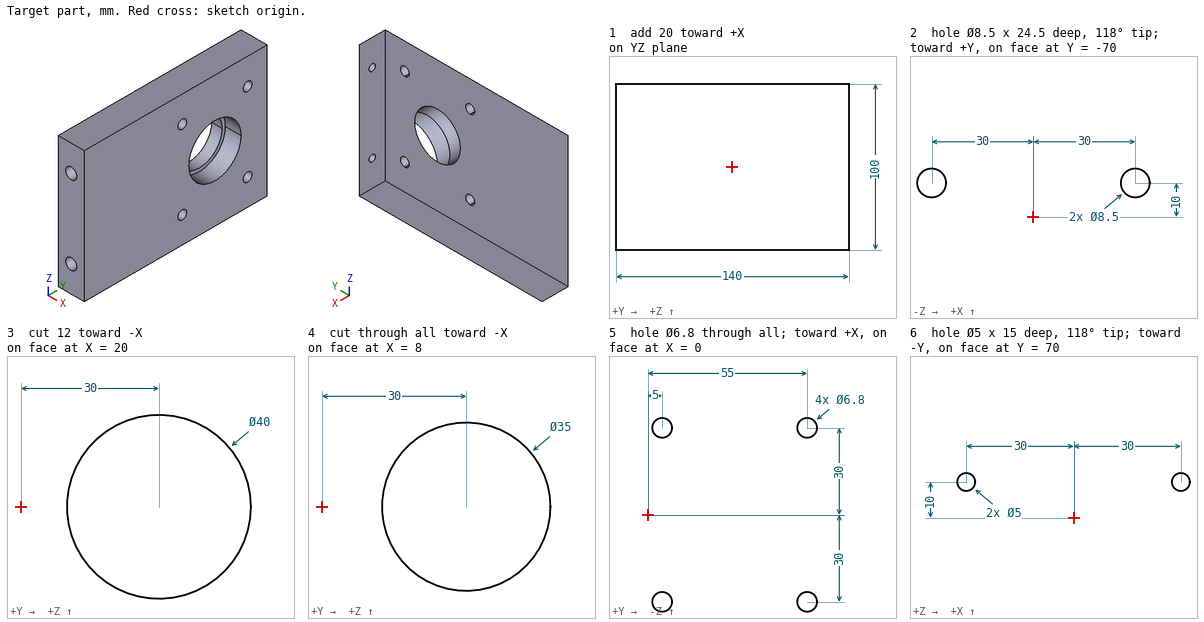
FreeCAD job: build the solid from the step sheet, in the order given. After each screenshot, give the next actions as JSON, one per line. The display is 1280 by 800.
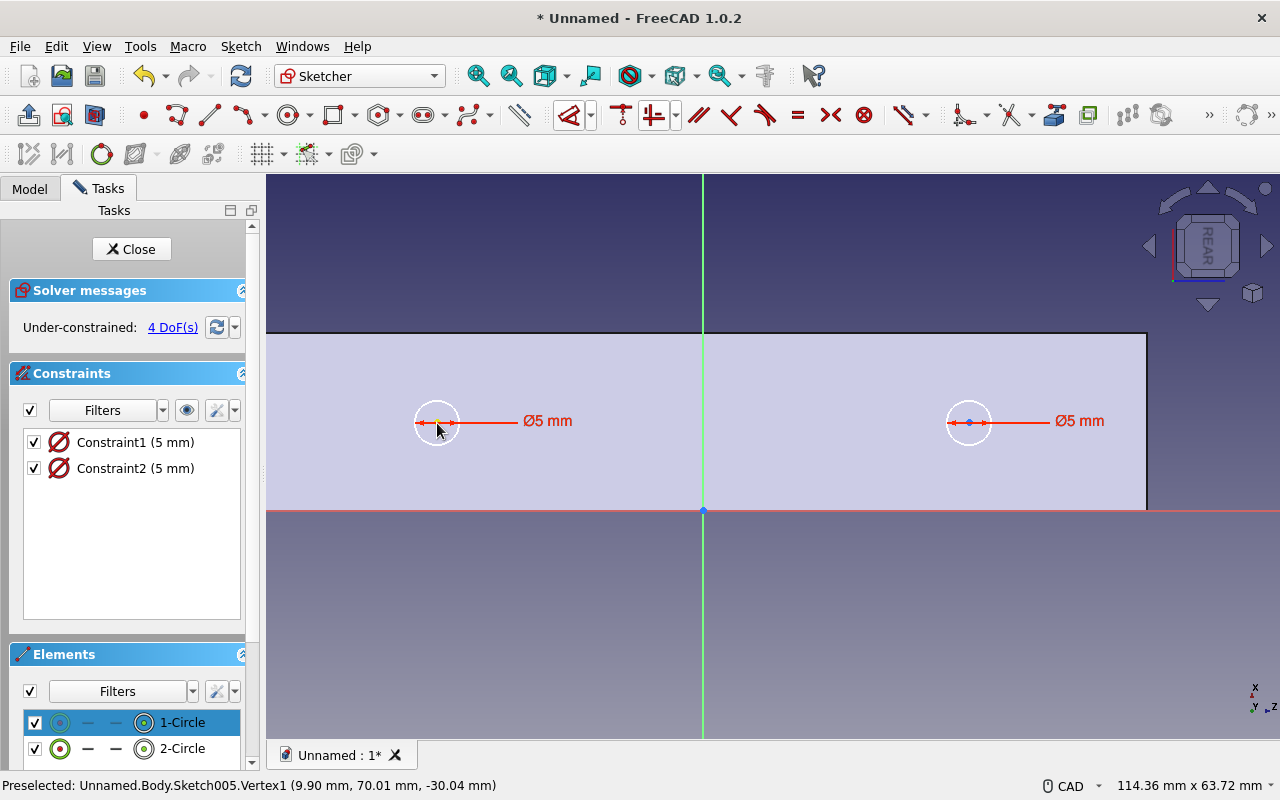
{"action": "left_click", "coordinate": [969, 423]}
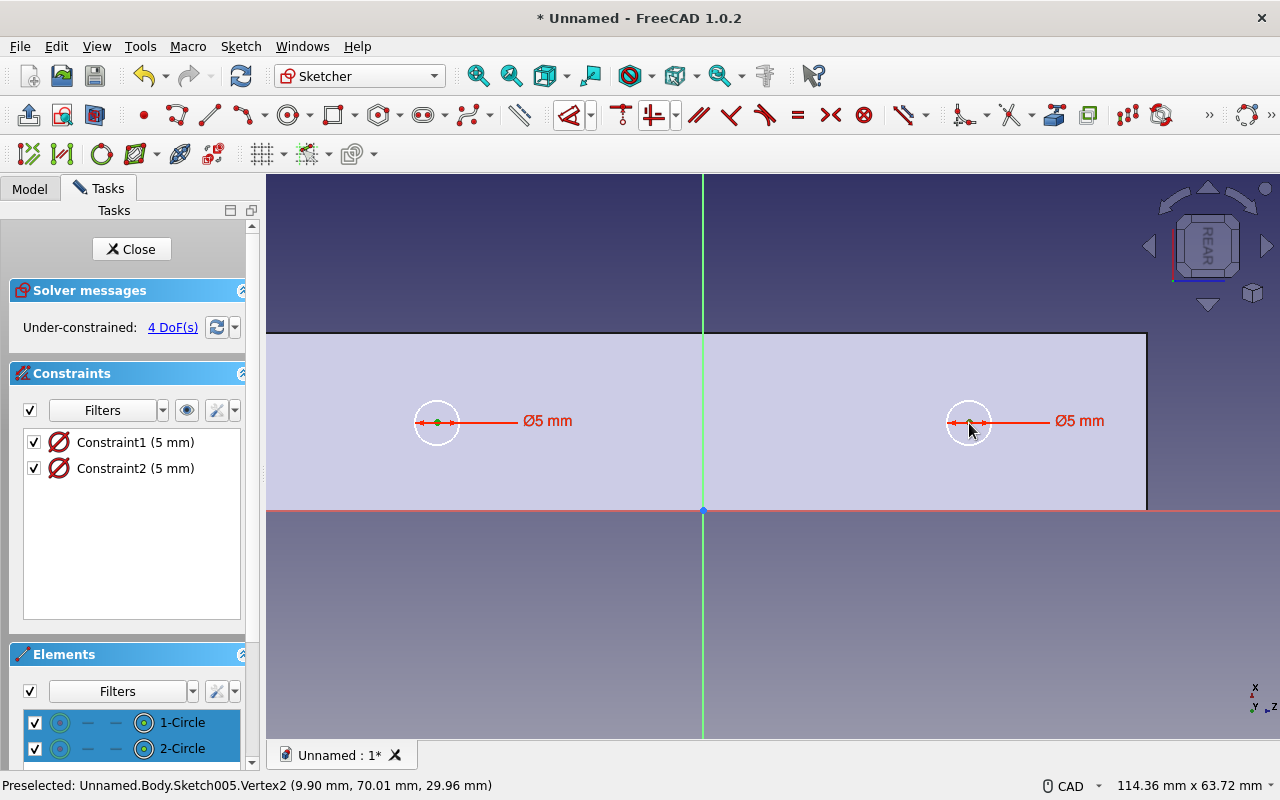
{"action": "key", "text": "h"}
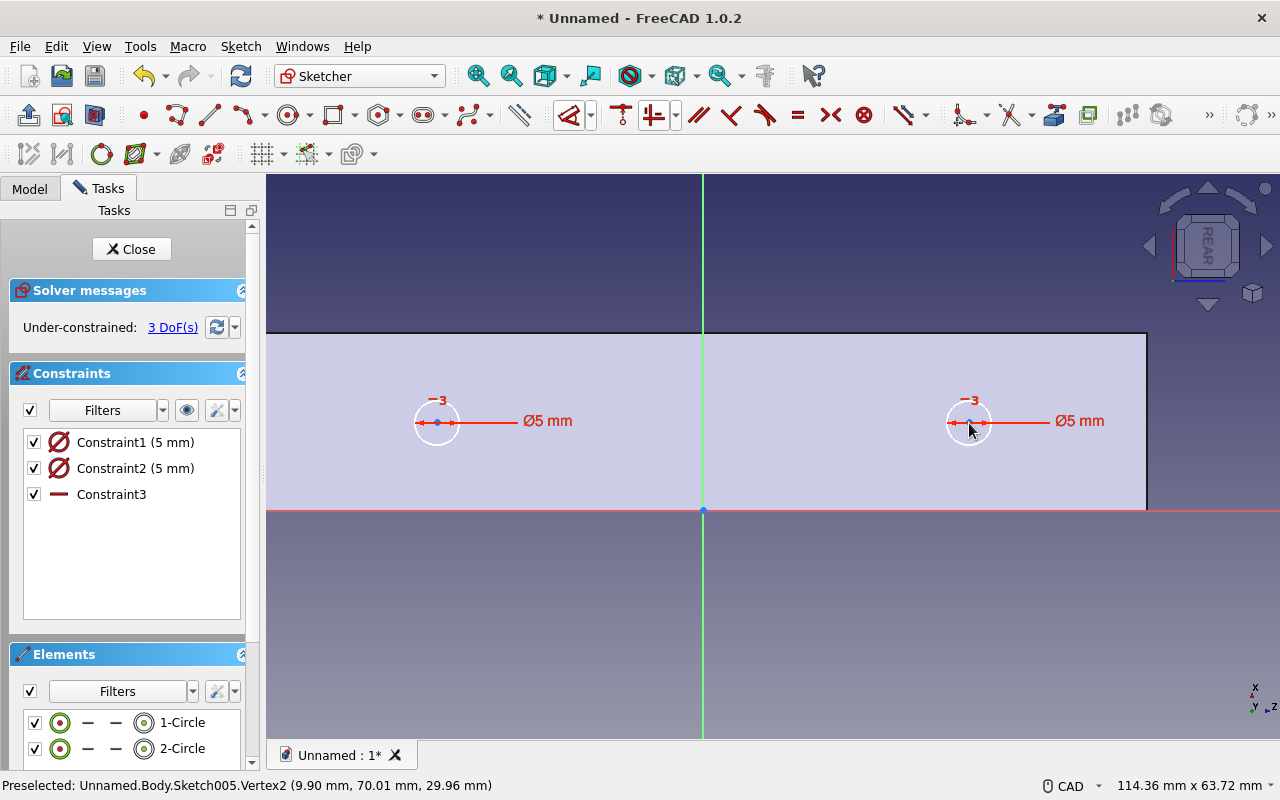
{"action": "left_click", "coordinate": [437, 423]}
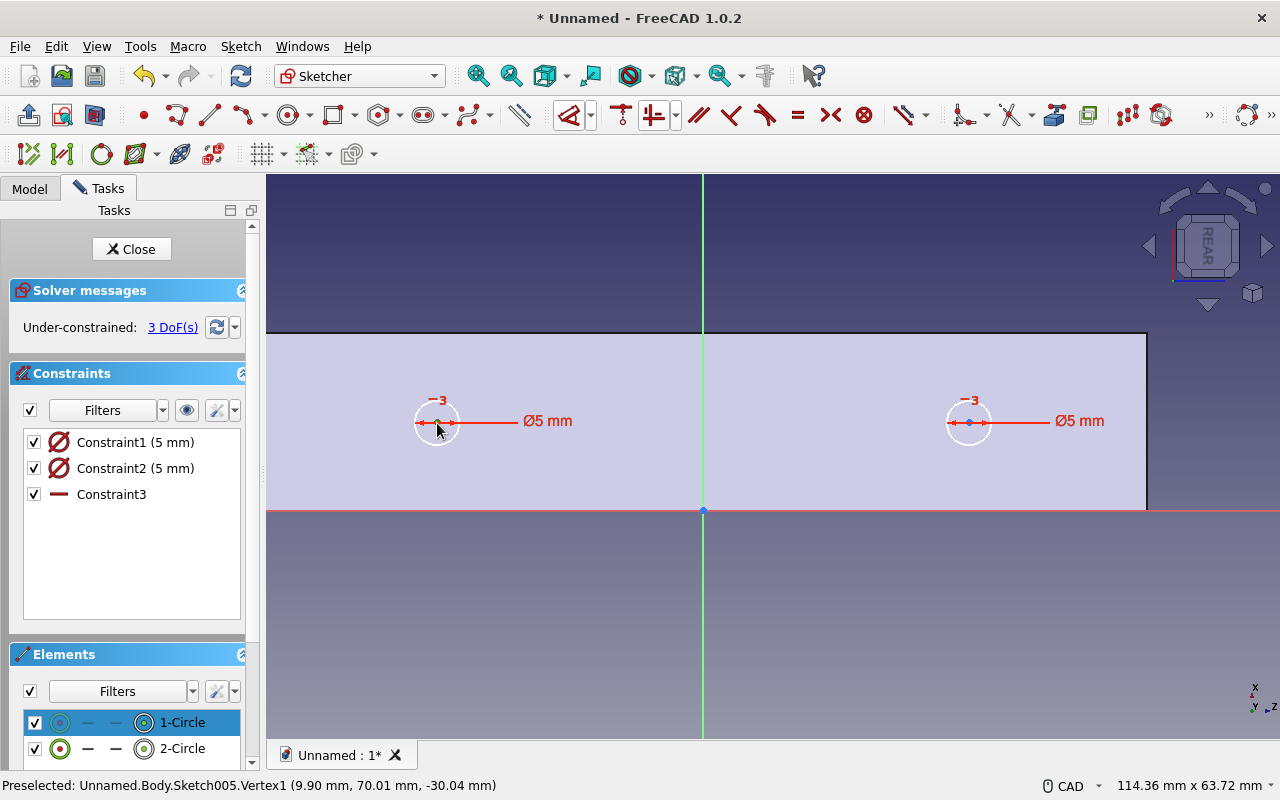
{"action": "key", "text": "l"}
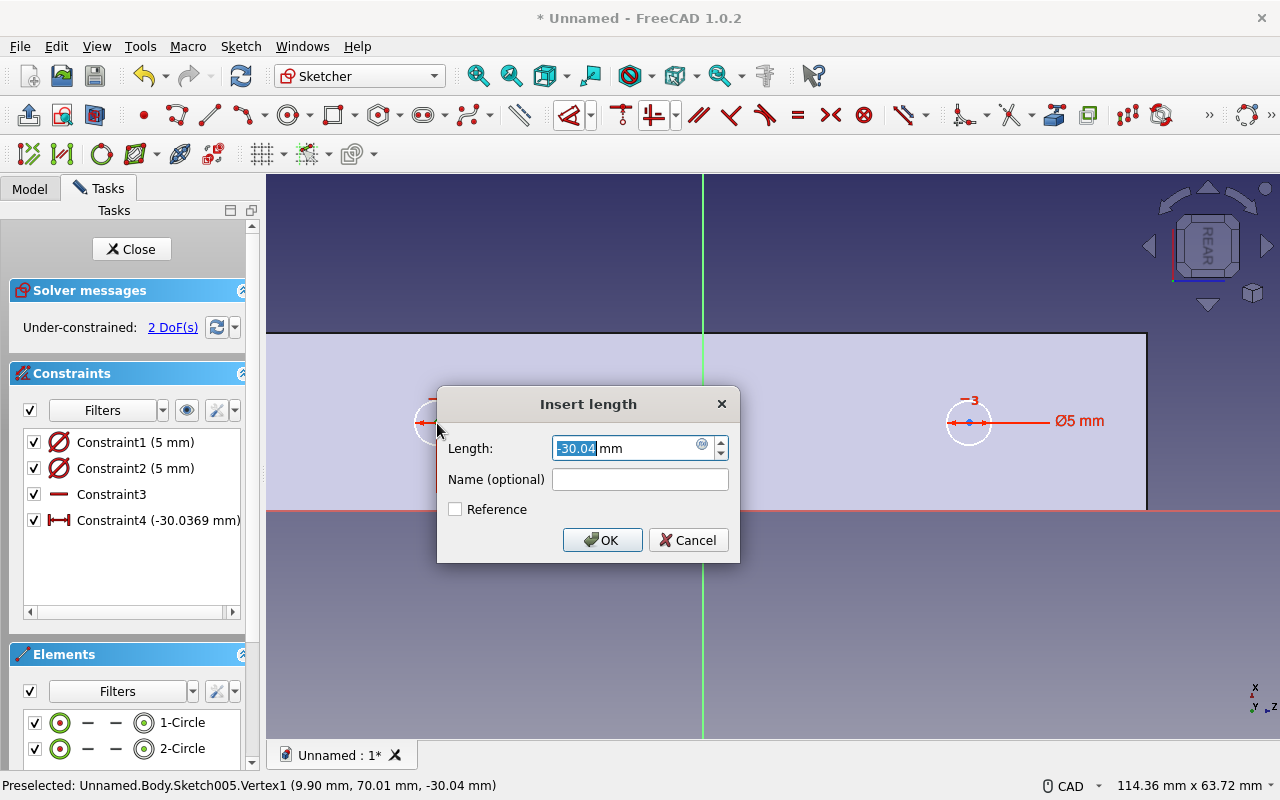
{"action": "type", "text": "-30"}
{"action": "key", "text": "Return"}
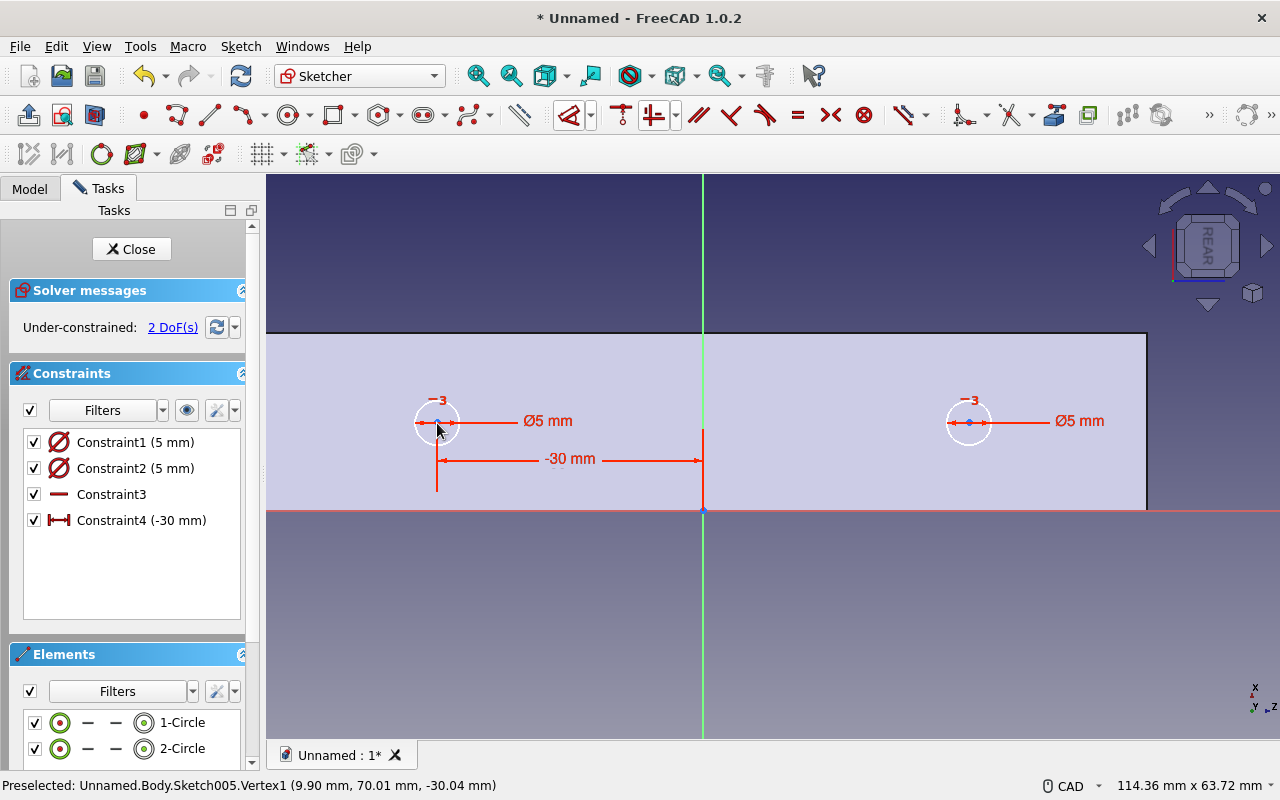
{"action": "left_click", "coordinate": [437, 423]}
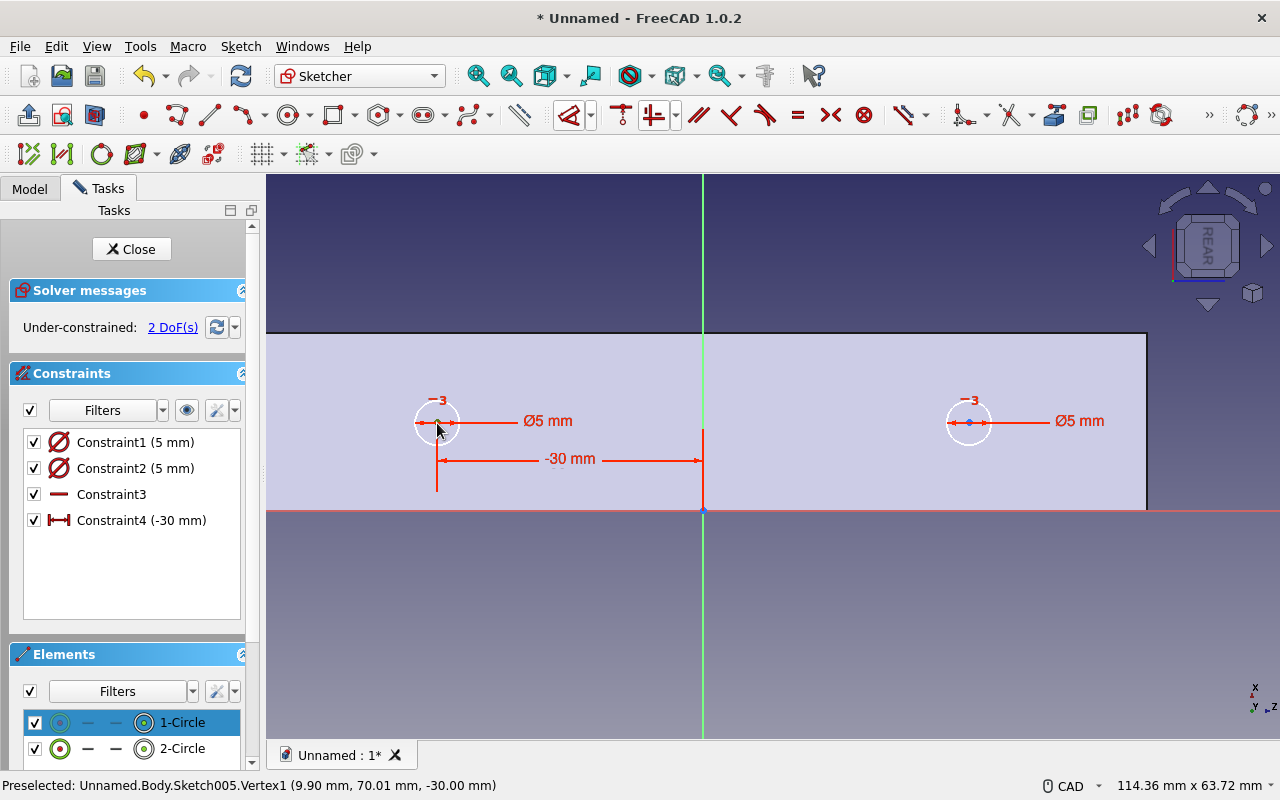
{"action": "key", "text": "i"}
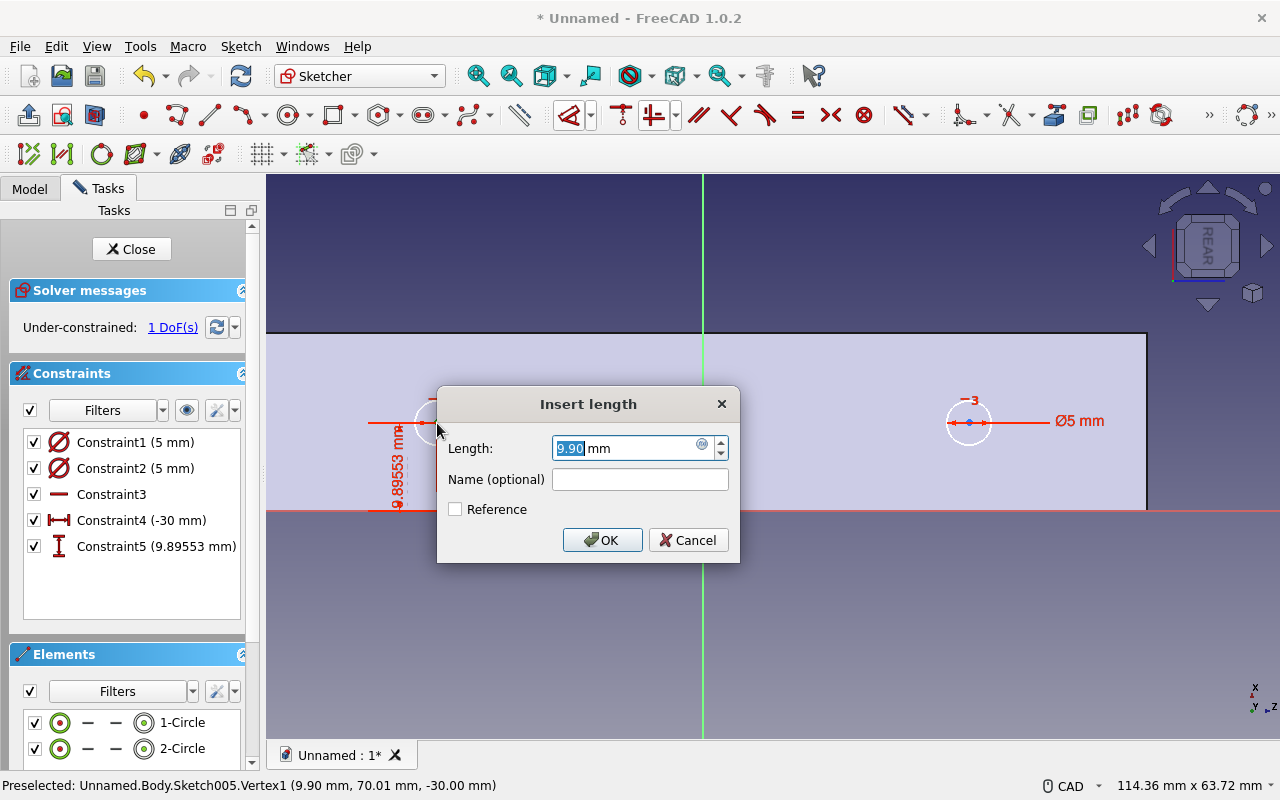
{"action": "type", "text": "10"}
{"action": "key", "text": "Return"}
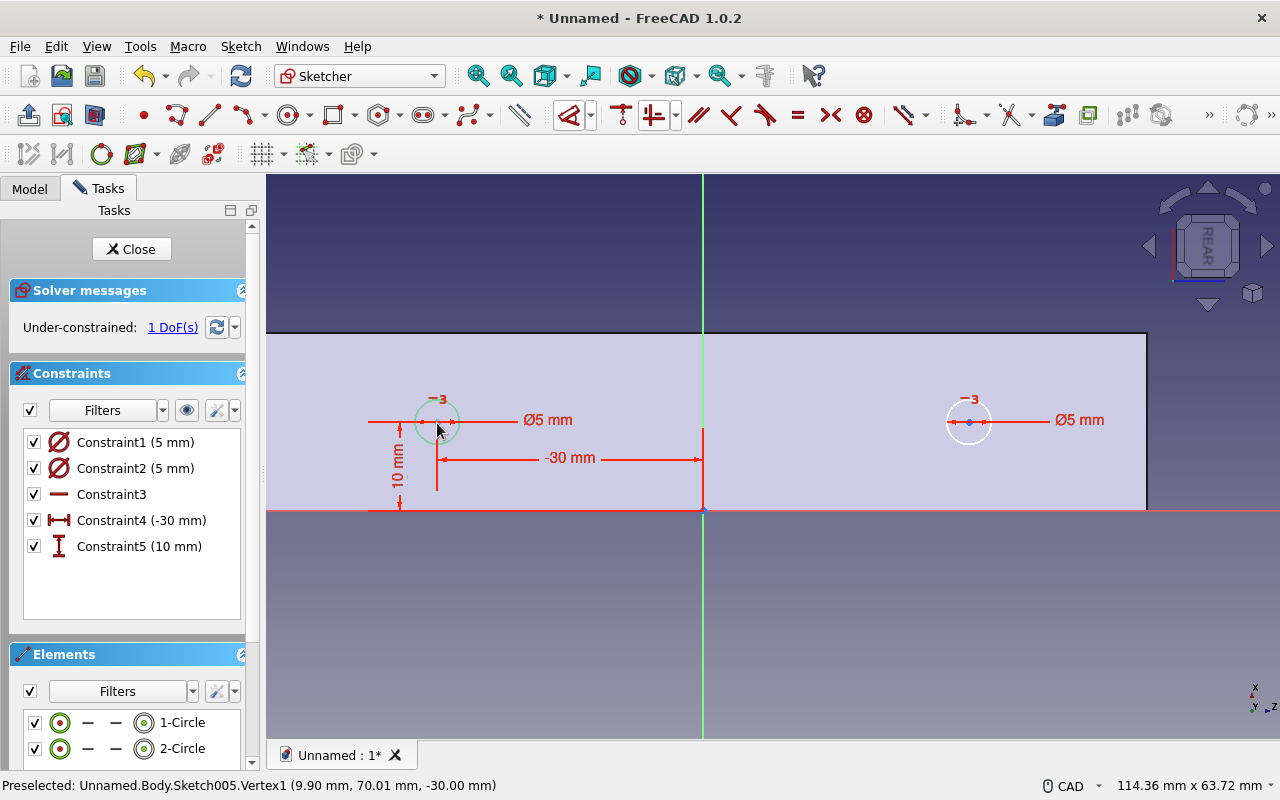
{"action": "left_click", "coordinate": [969, 422]}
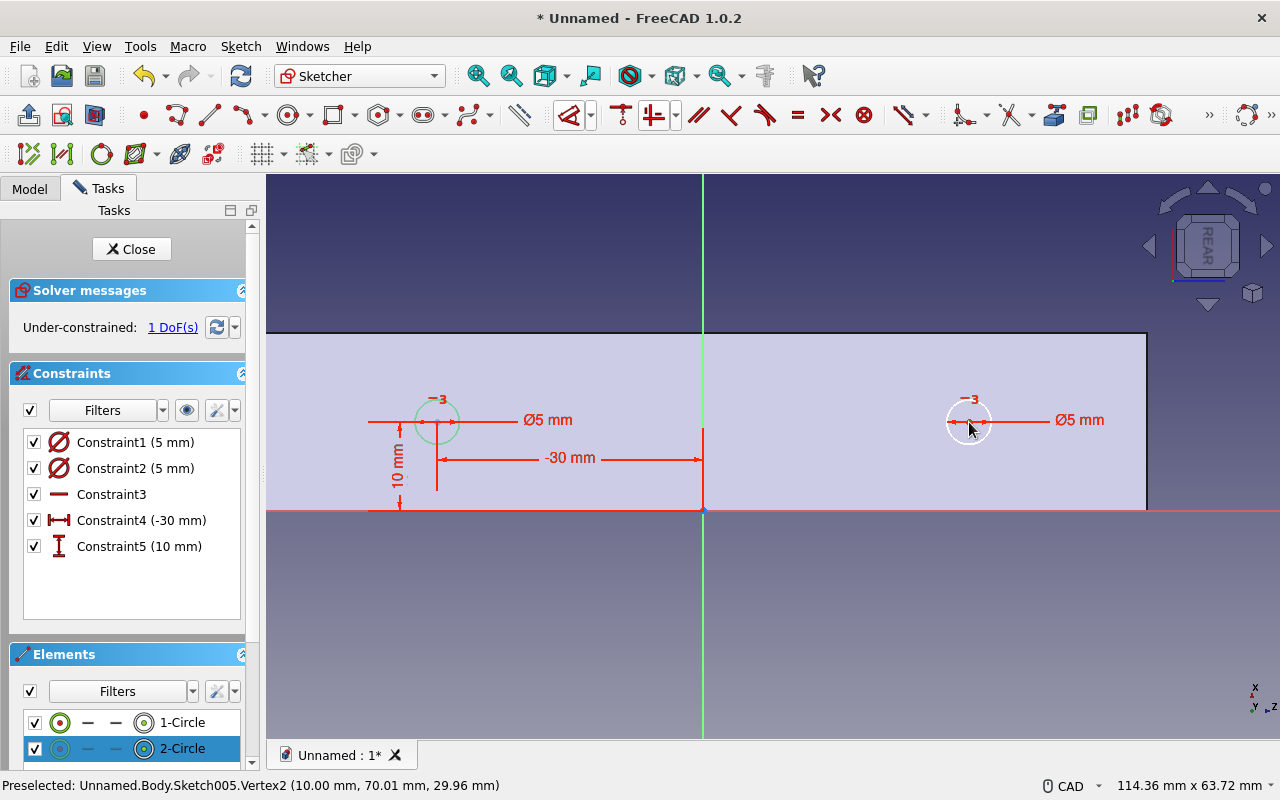
{"action": "left_click", "coordinate": [590, 116]}